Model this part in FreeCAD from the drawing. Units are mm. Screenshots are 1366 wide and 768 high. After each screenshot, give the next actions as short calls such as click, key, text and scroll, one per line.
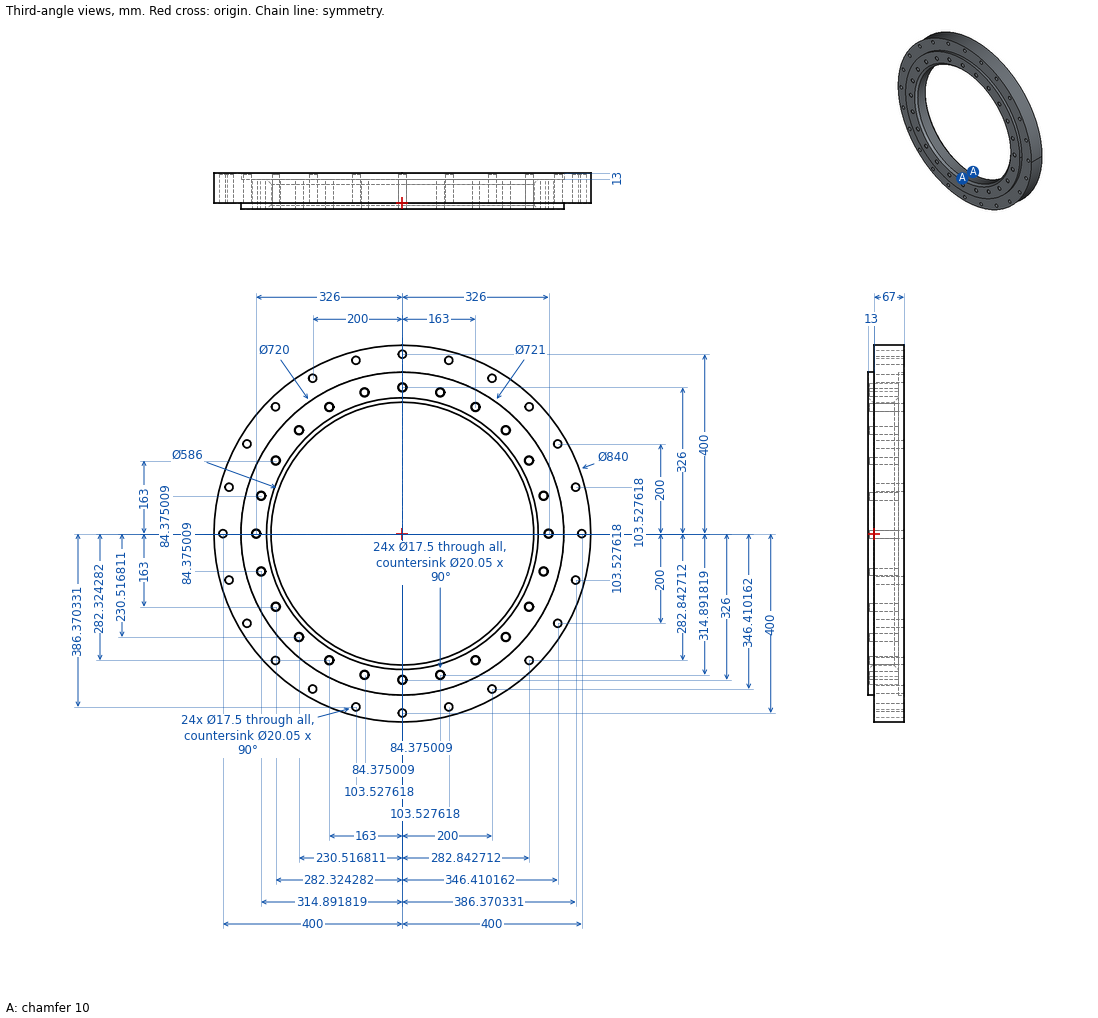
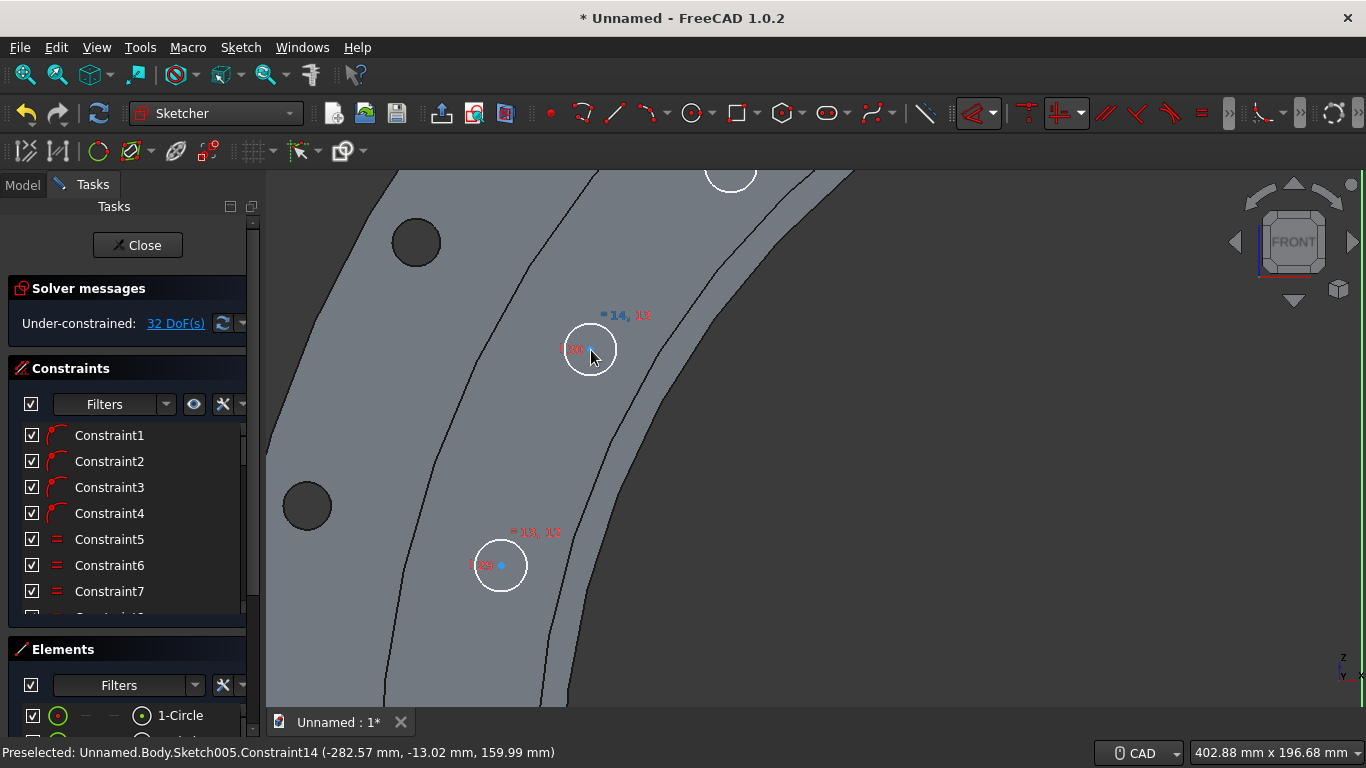
click(591, 349)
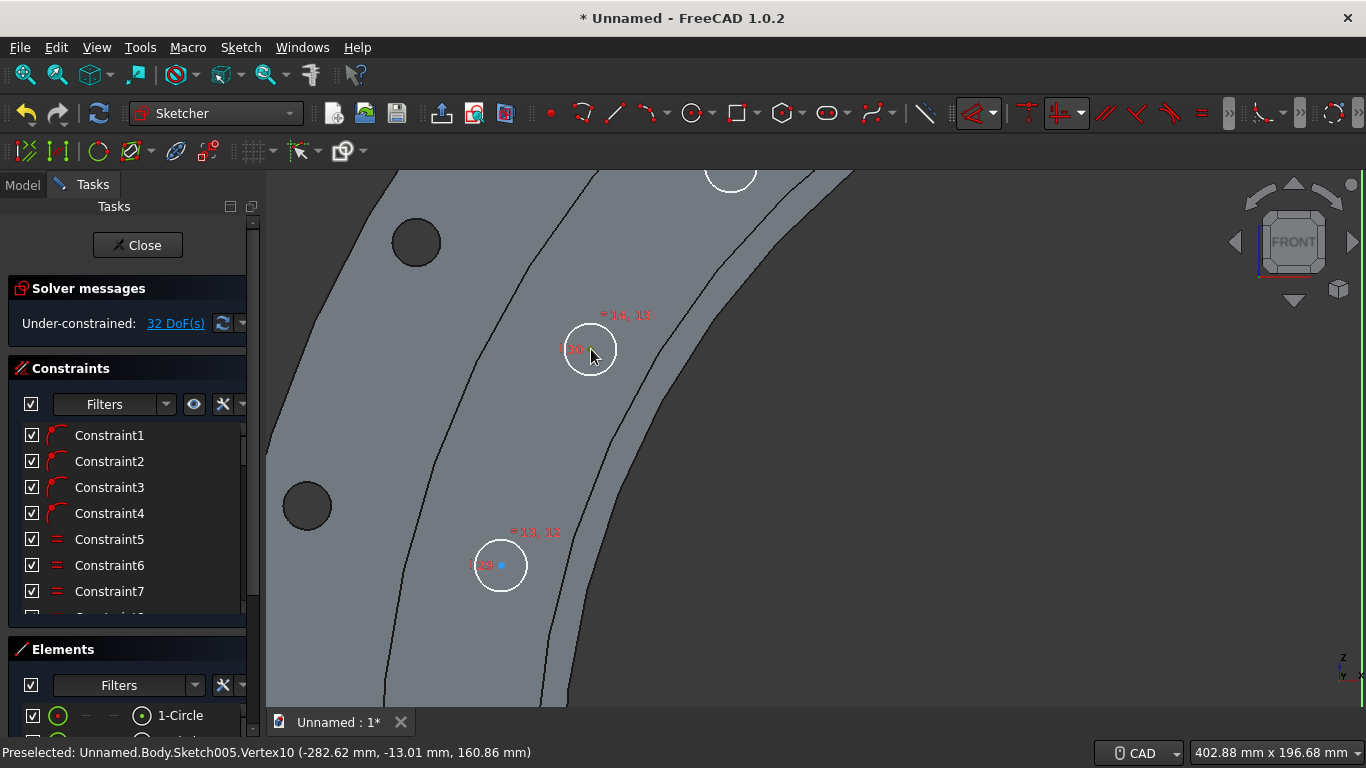
scroll(592, 350, down, 8)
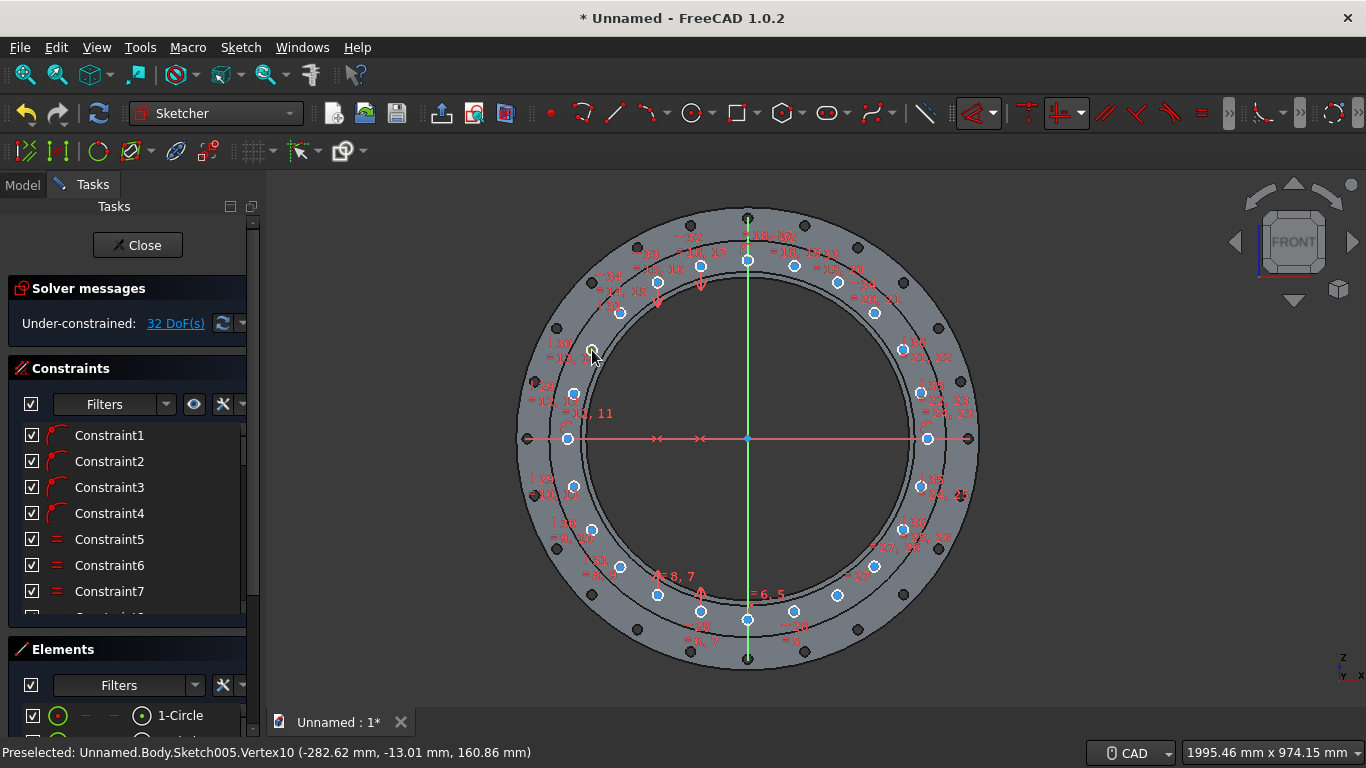
click(903, 350)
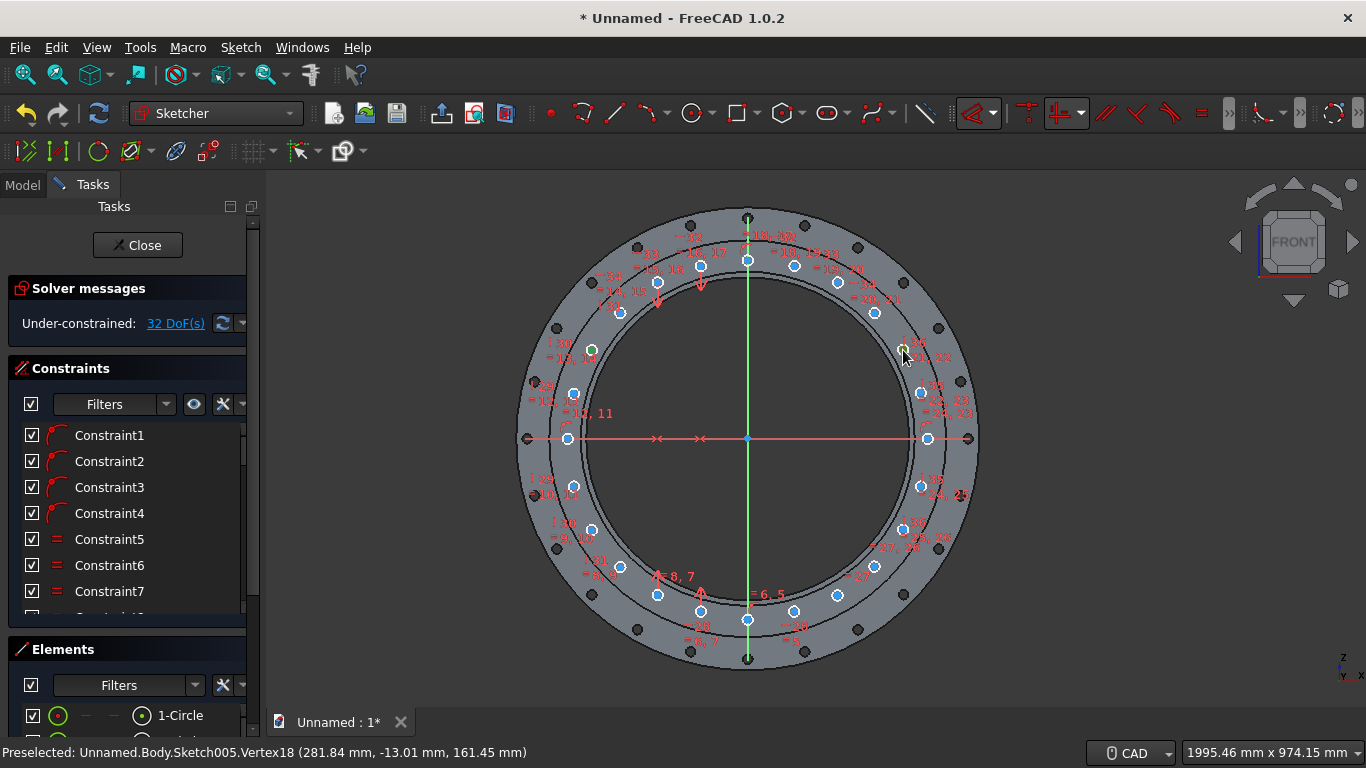
click(748, 576)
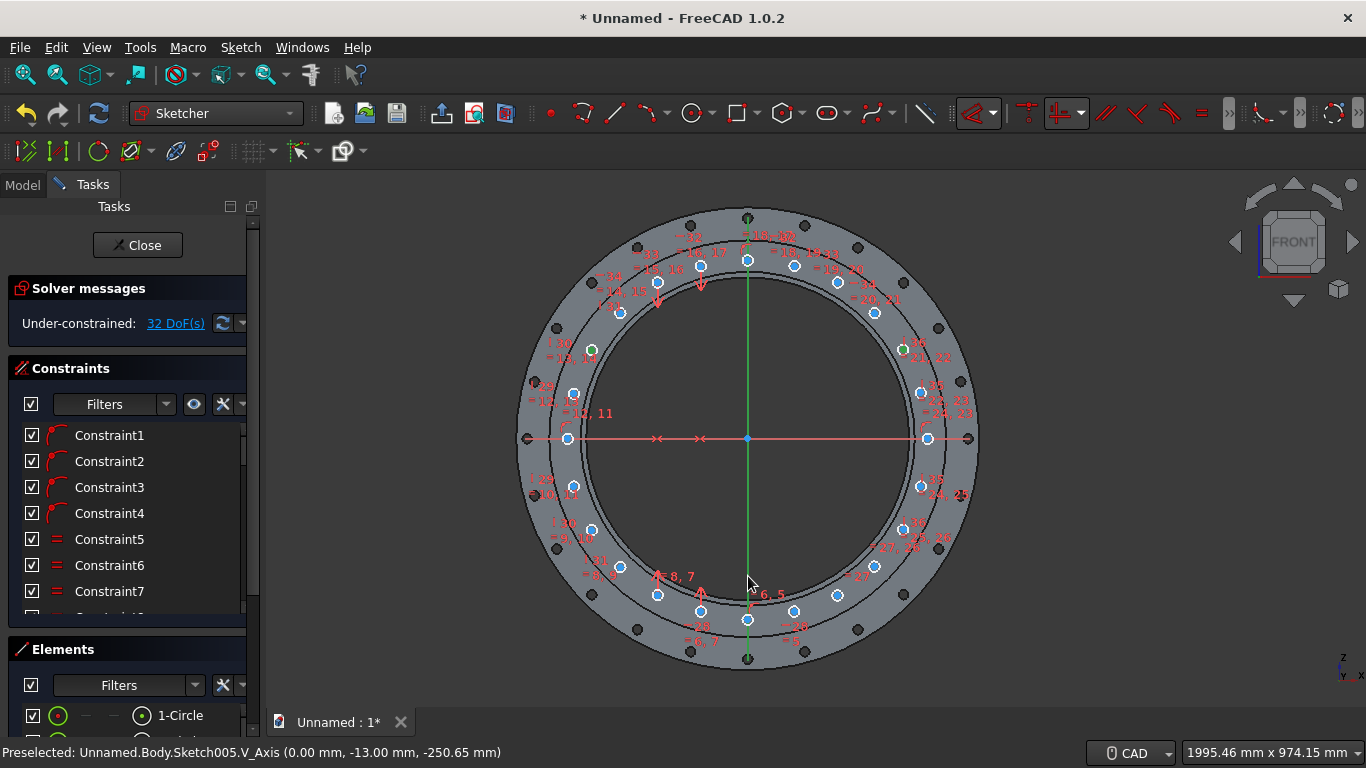
key(s)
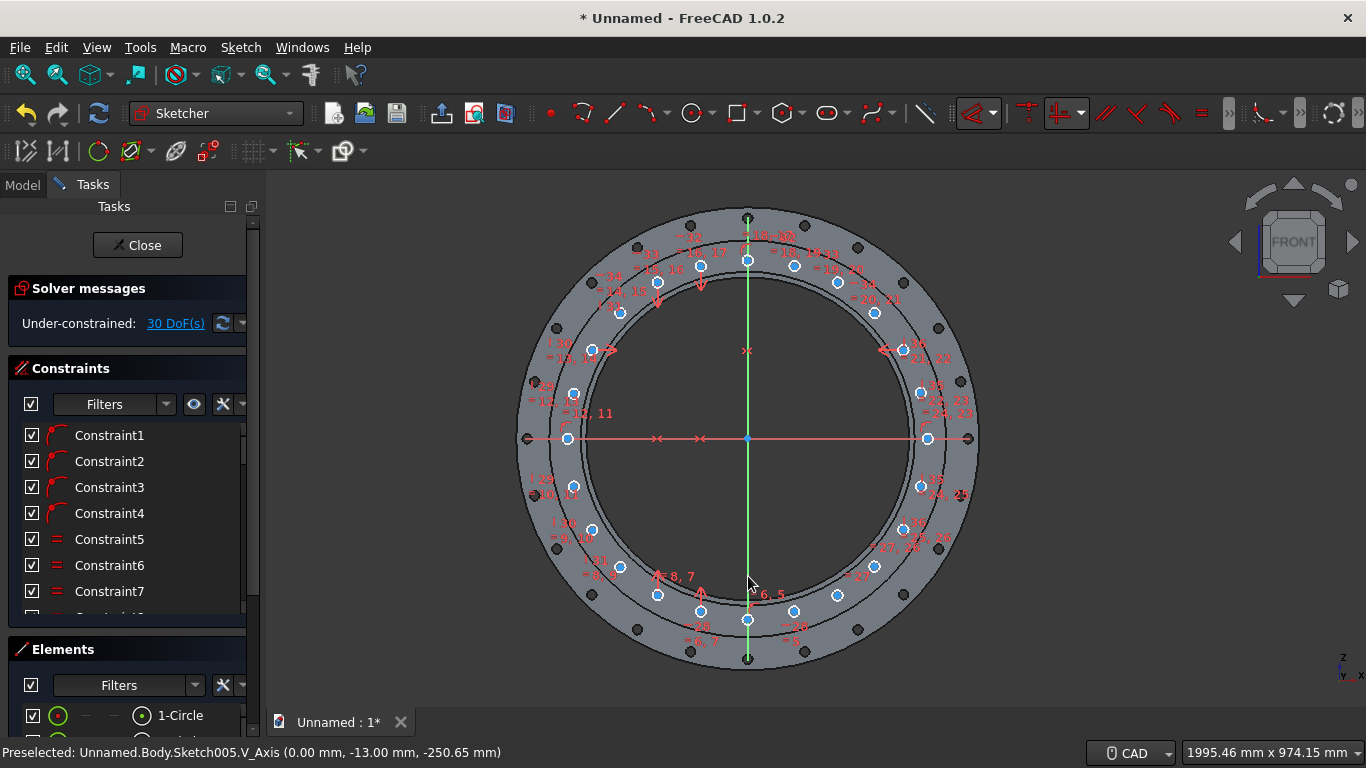
scroll(574, 394, up, 4)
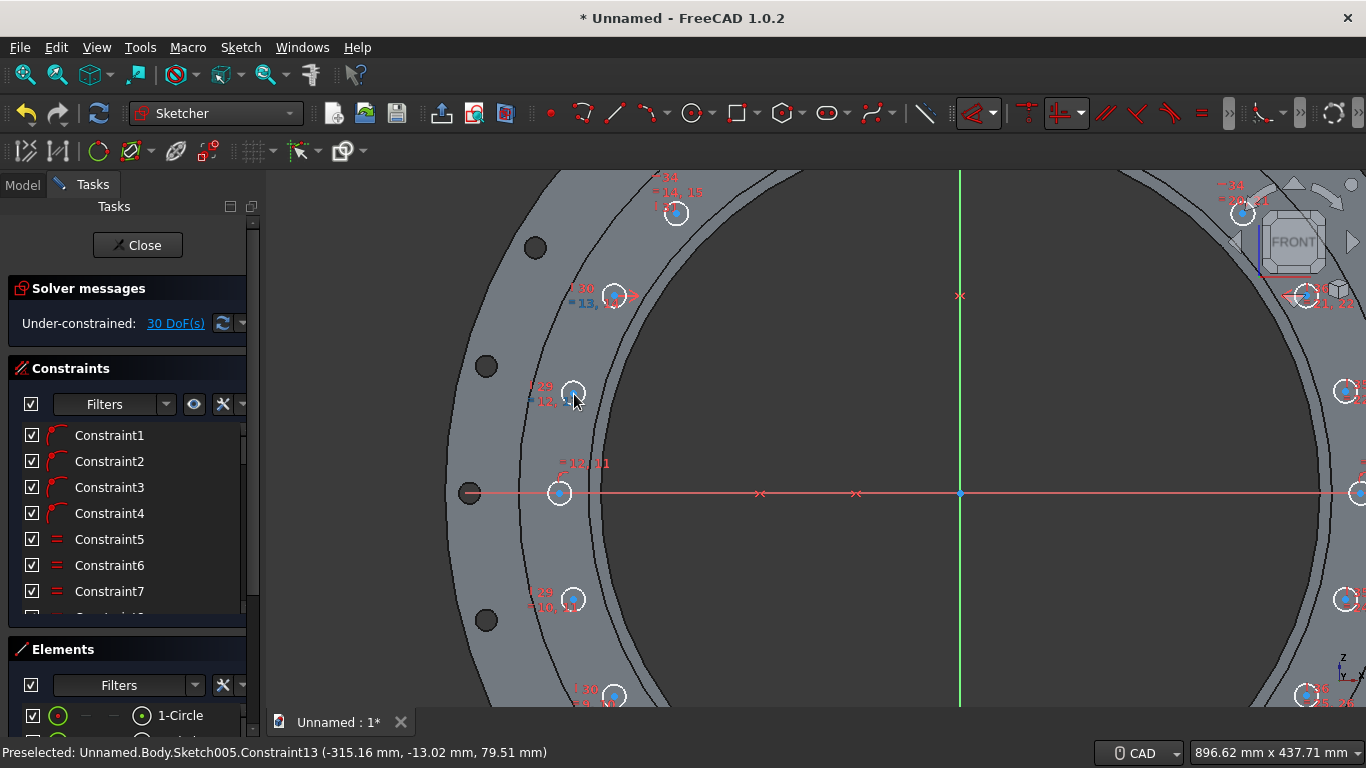
scroll(573, 393, up, 4)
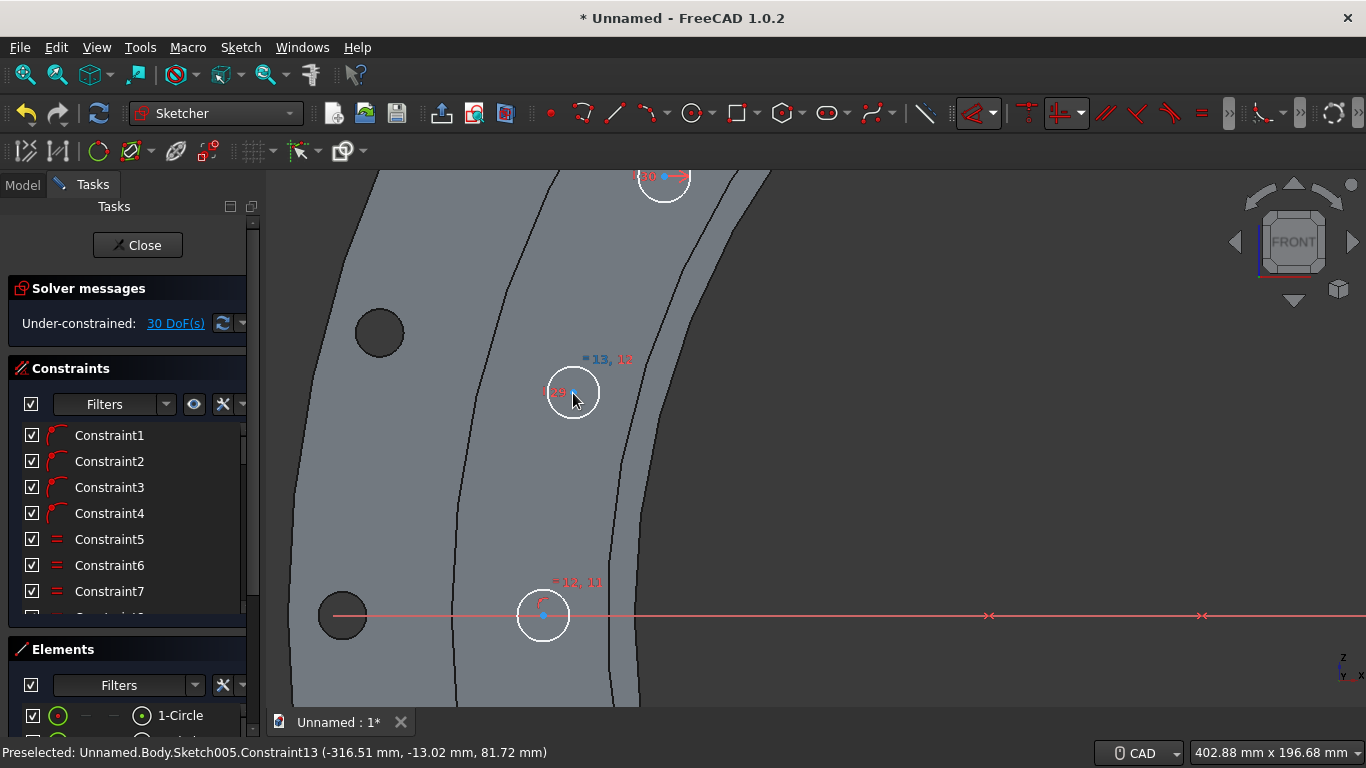
click(573, 393)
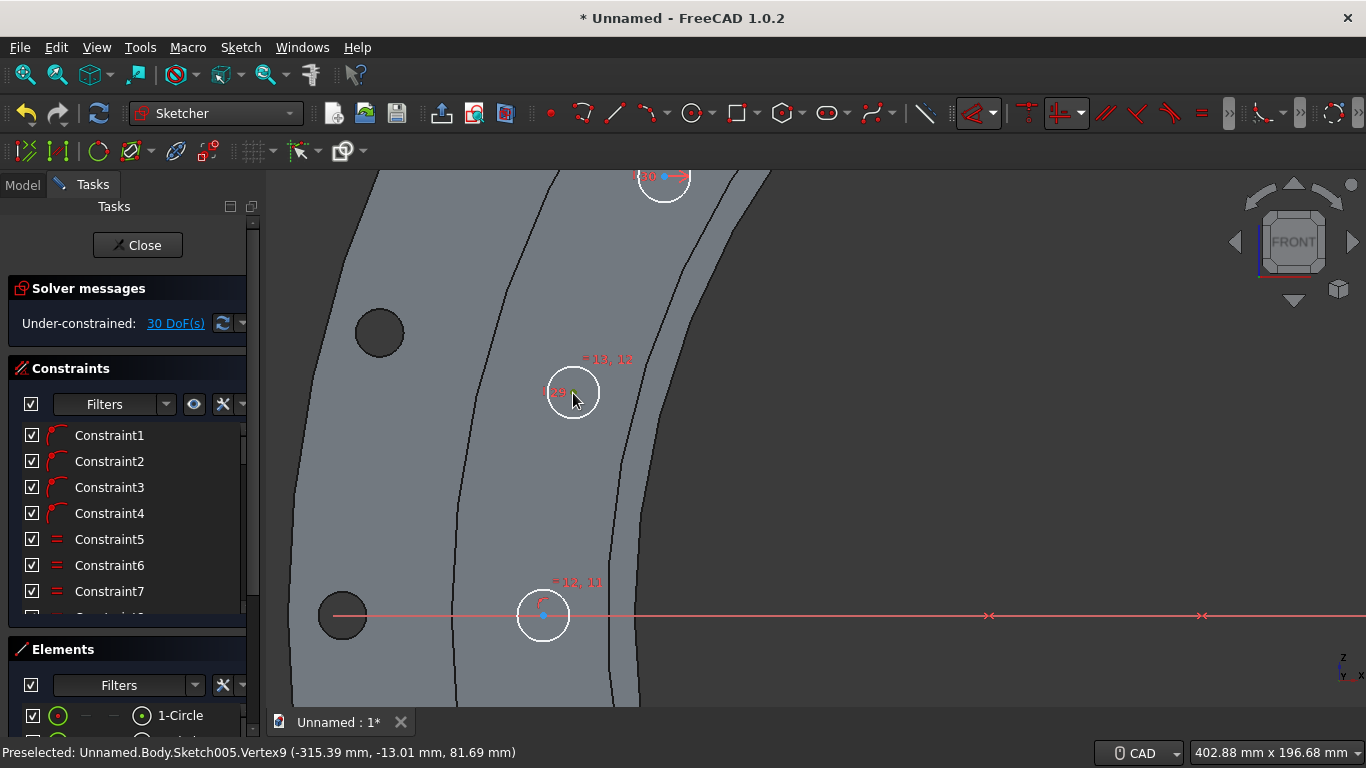
scroll(574, 394, down, 8)